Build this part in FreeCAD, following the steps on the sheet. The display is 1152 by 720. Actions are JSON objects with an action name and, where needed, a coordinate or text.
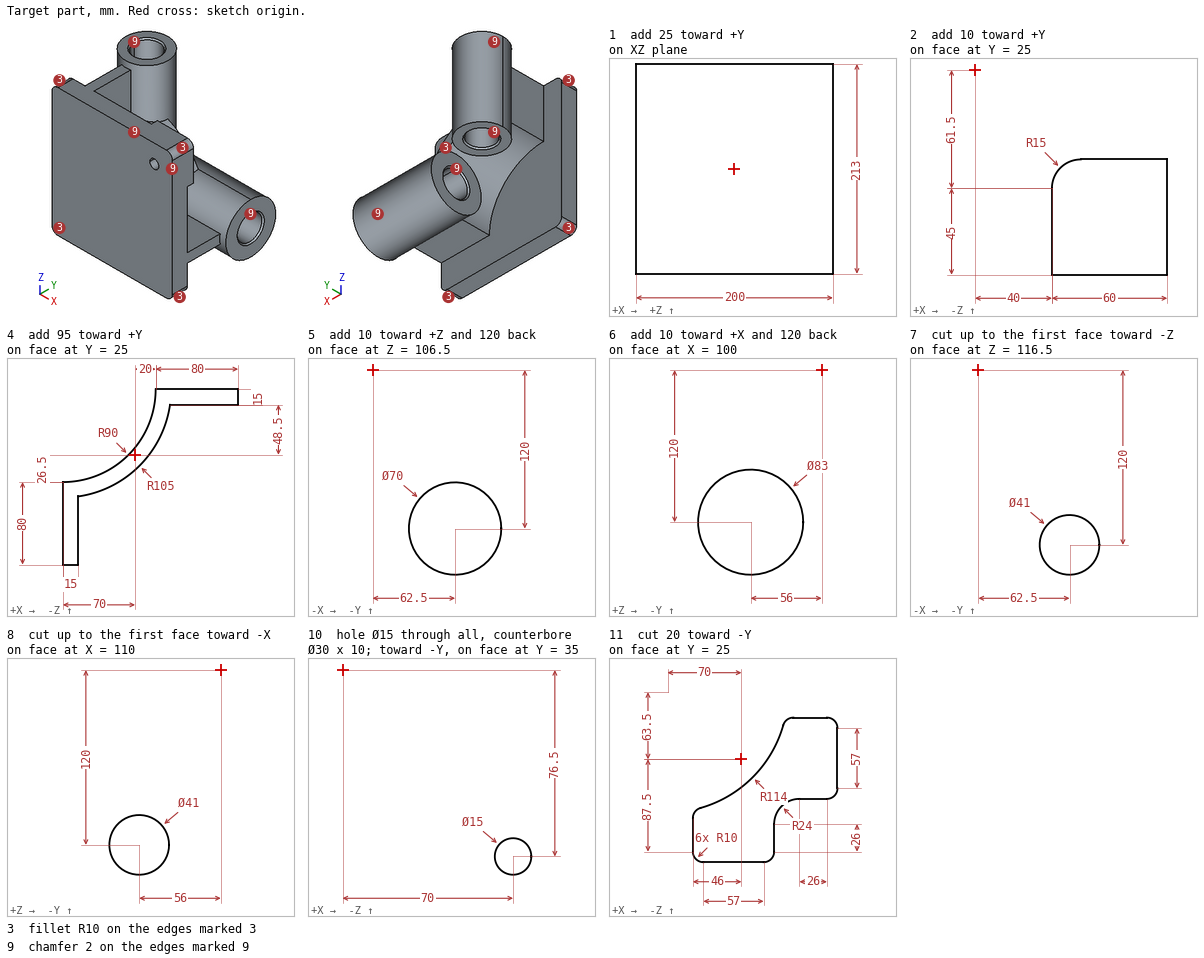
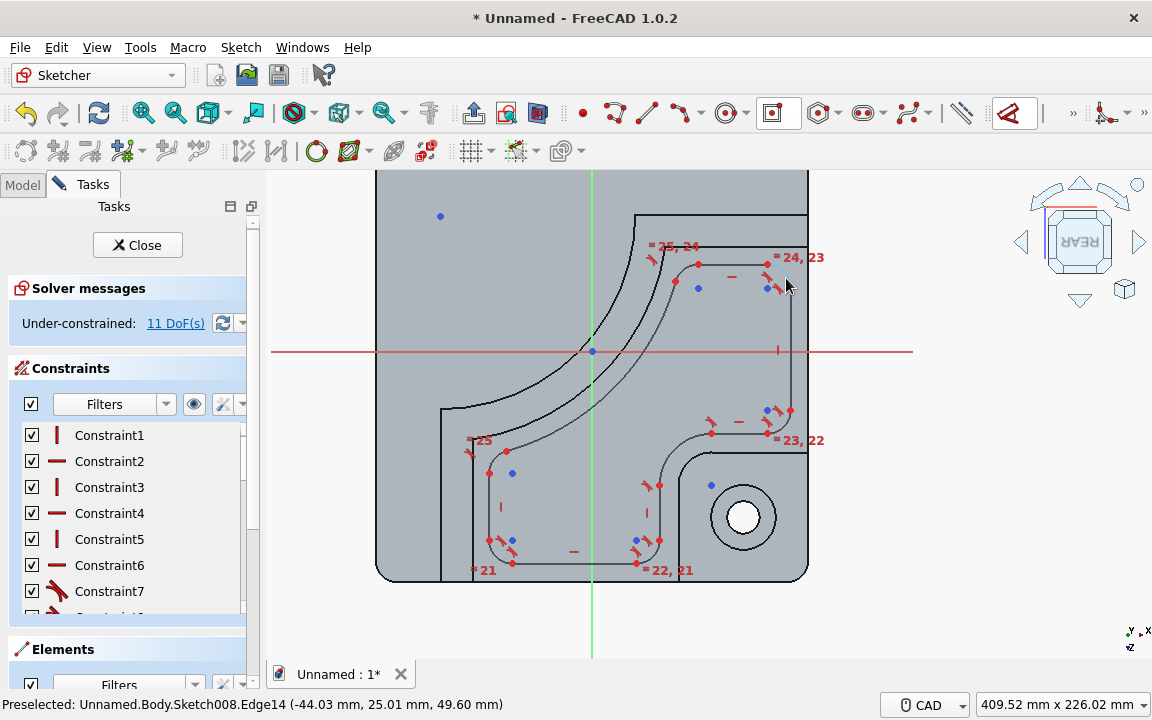
{"action": "scroll", "coordinate": [492, 551], "scroll_direction": "up", "scroll_amount": 4}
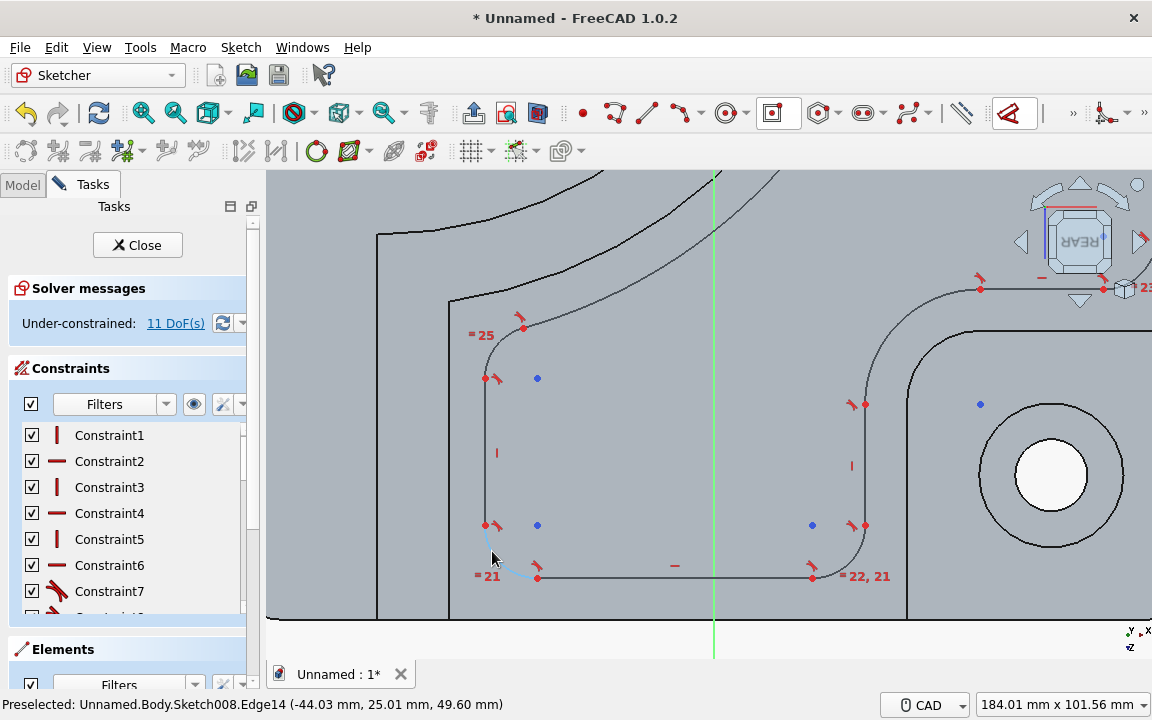
{"action": "left_click", "coordinate": [491, 549]}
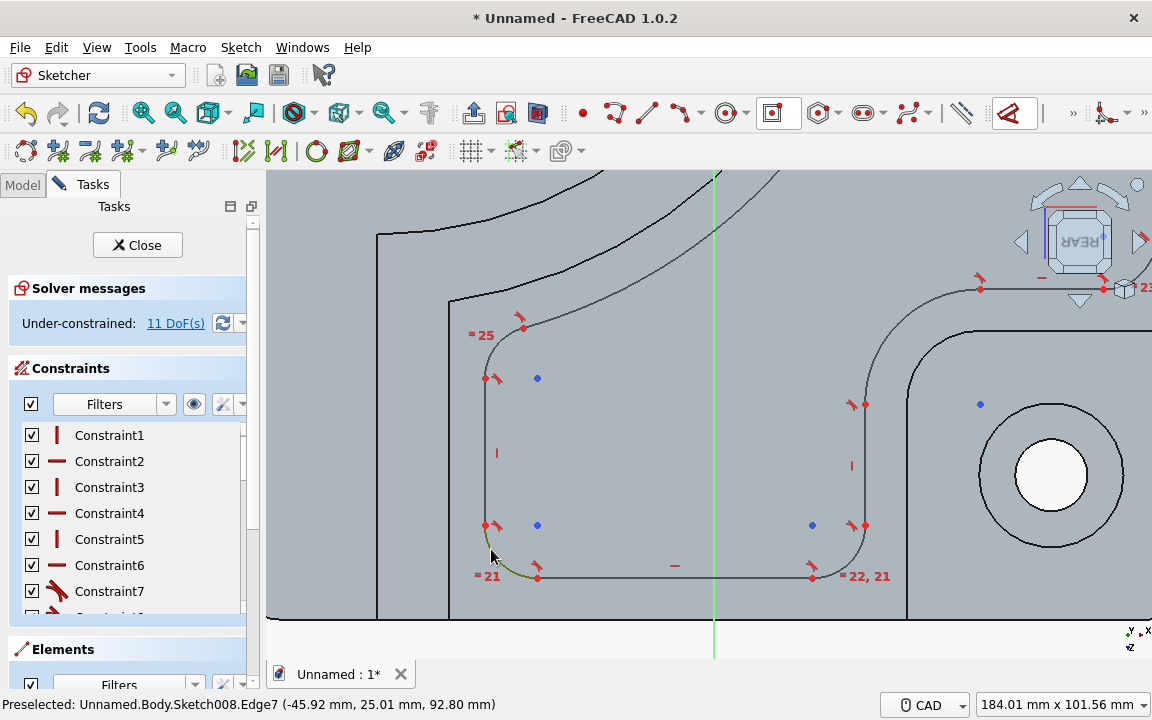
{"action": "key", "text": "k r"}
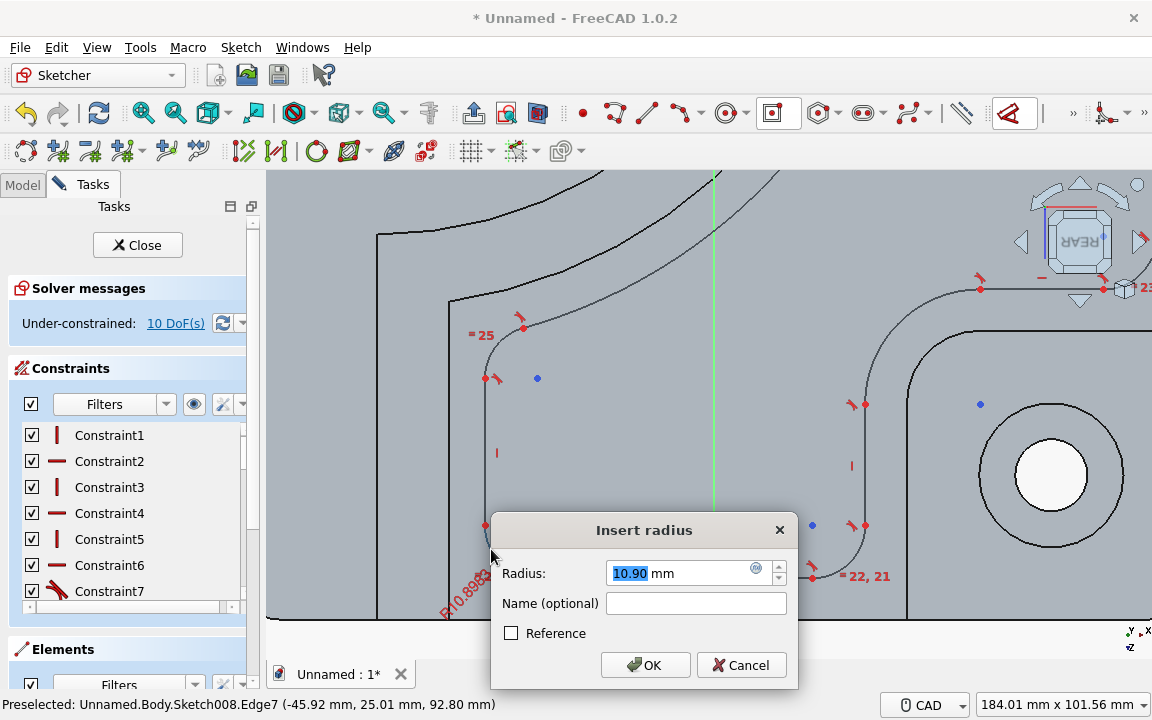
{"action": "type", "text": "10"}
{"action": "key", "text": "Return"}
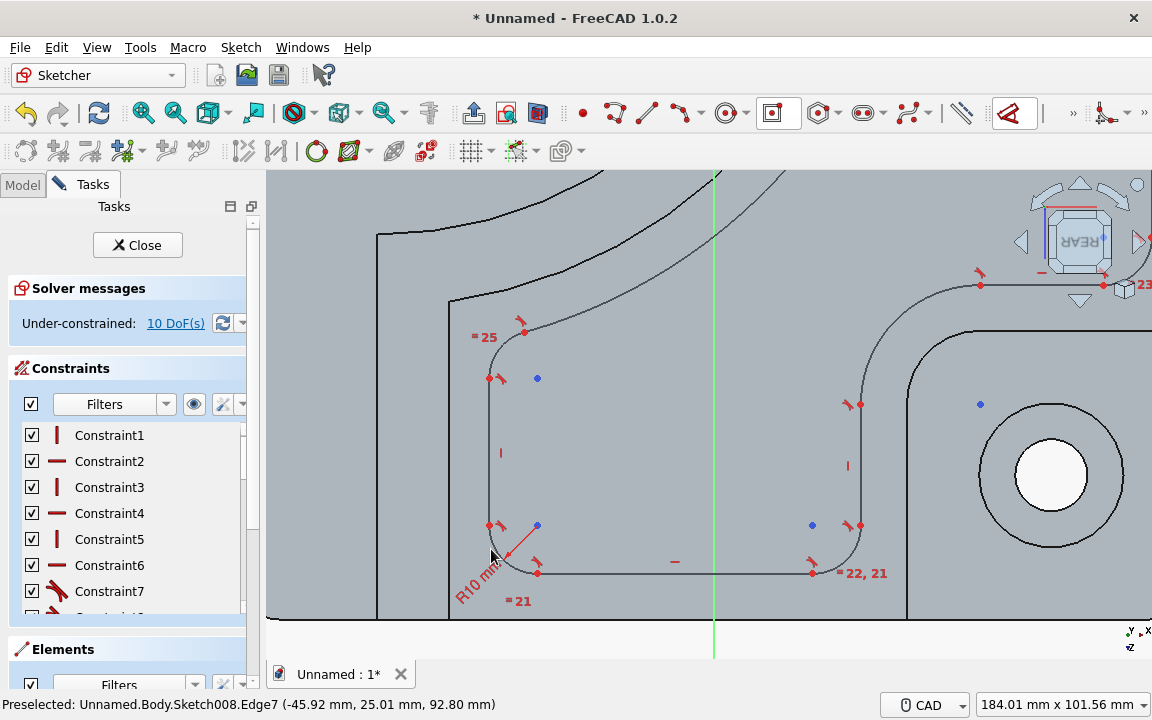
{"action": "left_click", "coordinate": [926, 298]}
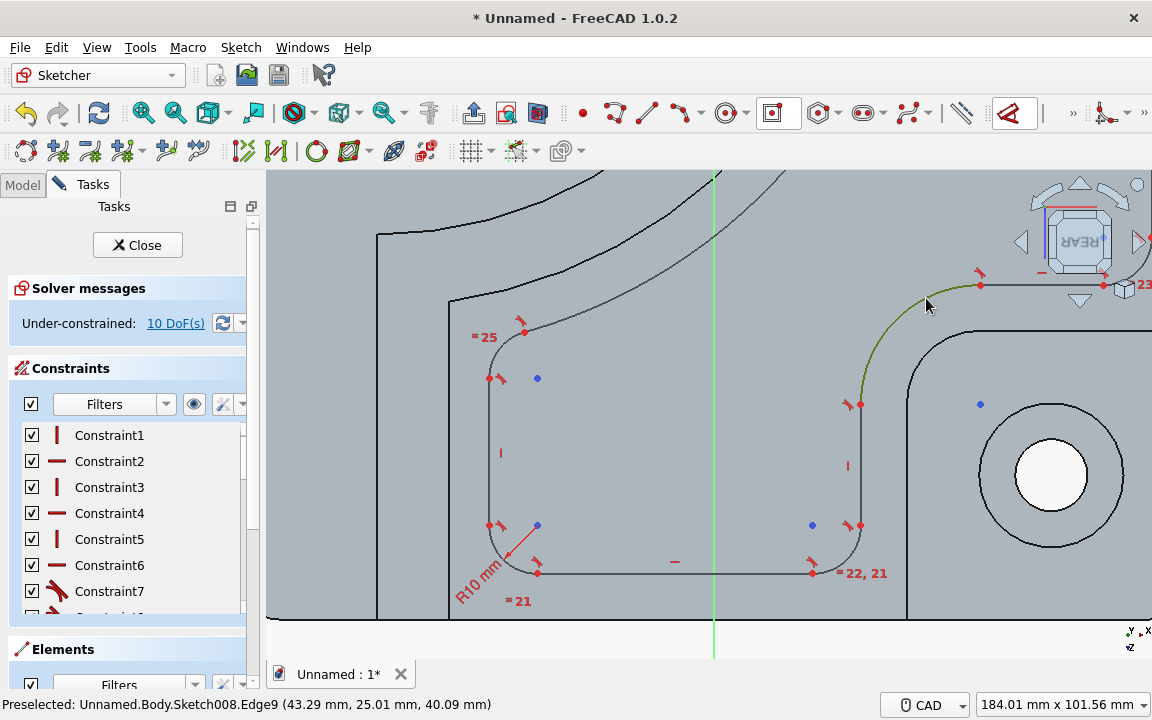
{"action": "left_click", "coordinate": [1032, 114]}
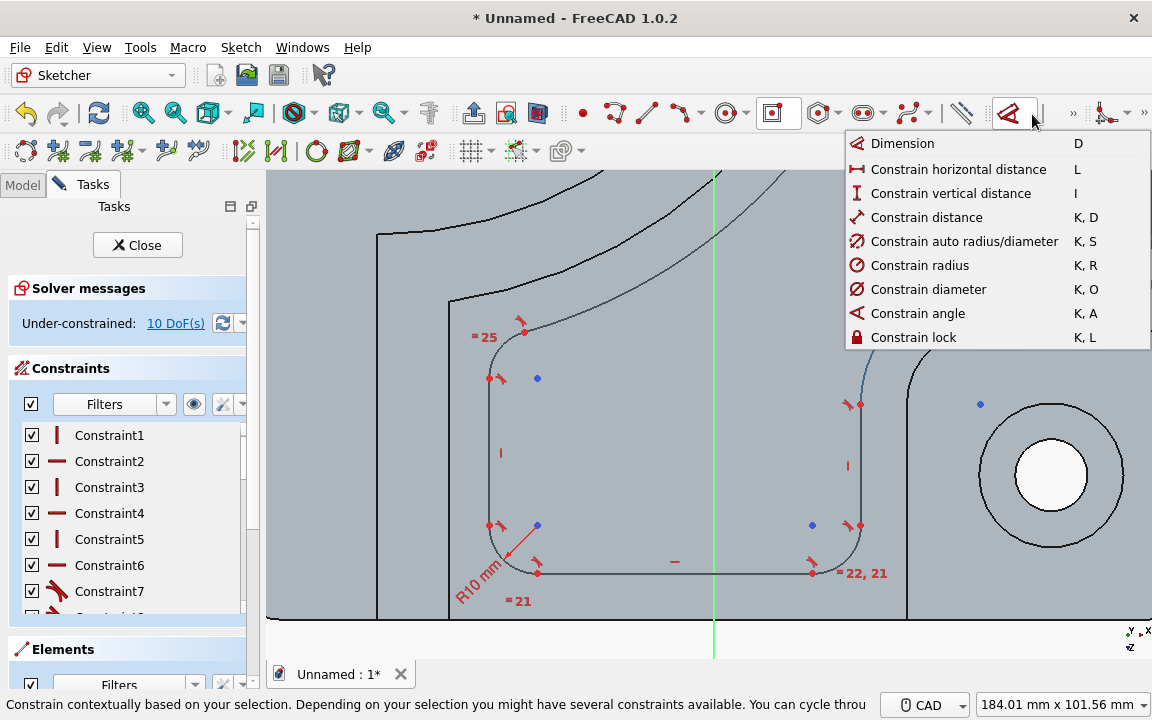
{"action": "left_click", "coordinate": [998, 265]}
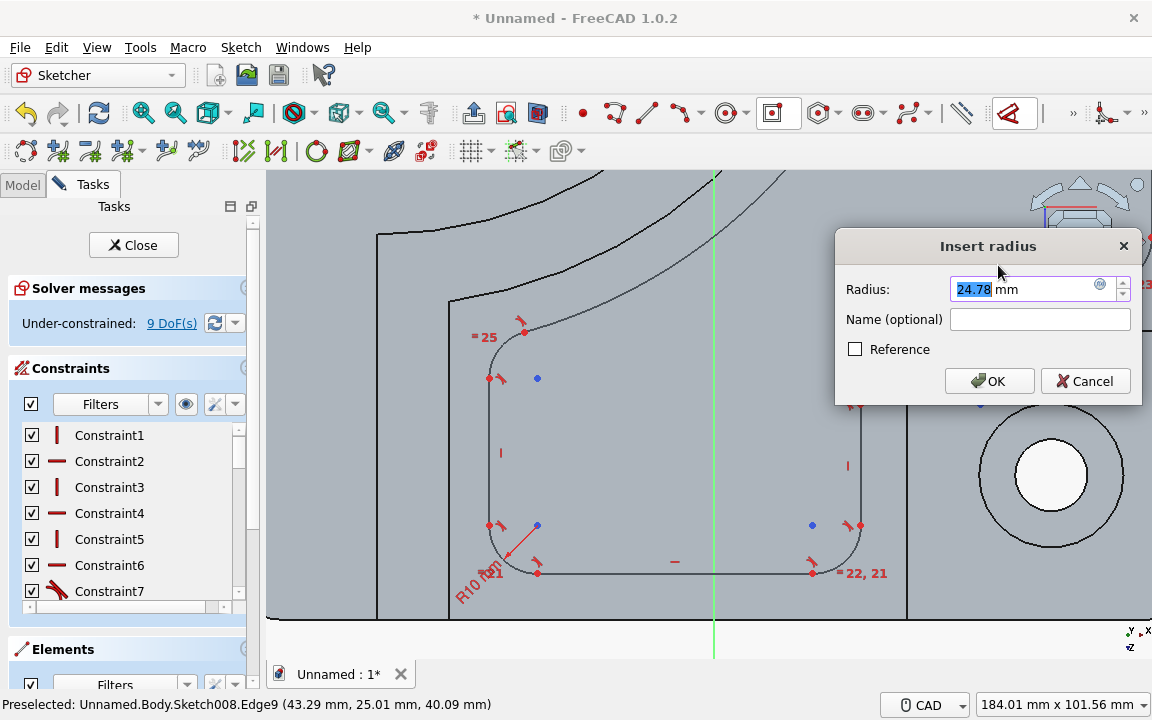
{"action": "type", "text": "24"}
{"action": "key", "text": "Return"}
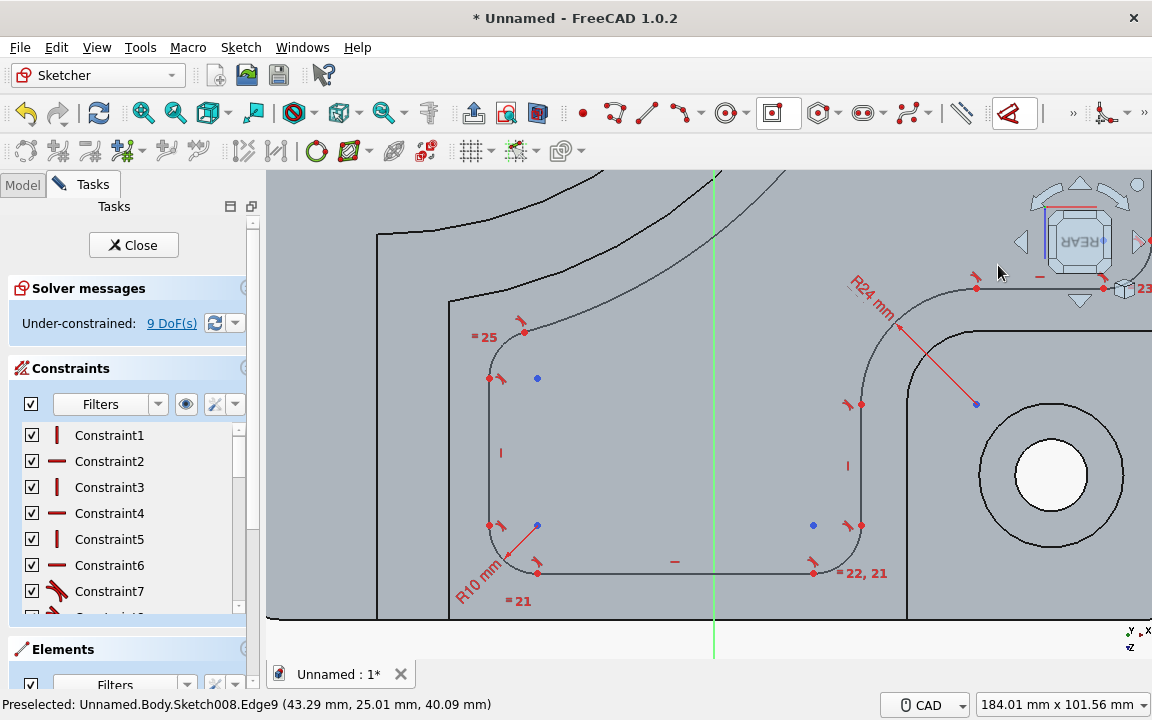
{"action": "left_click", "coordinate": [678, 263]}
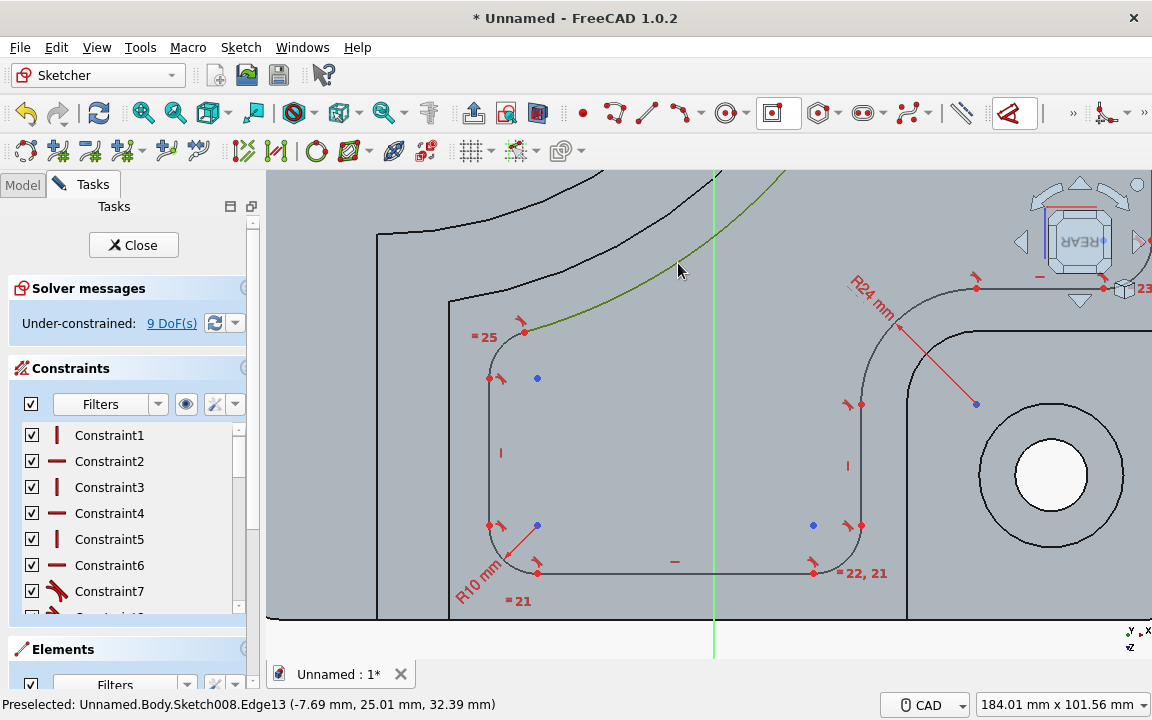
{"action": "left_click", "coordinate": [1032, 114]}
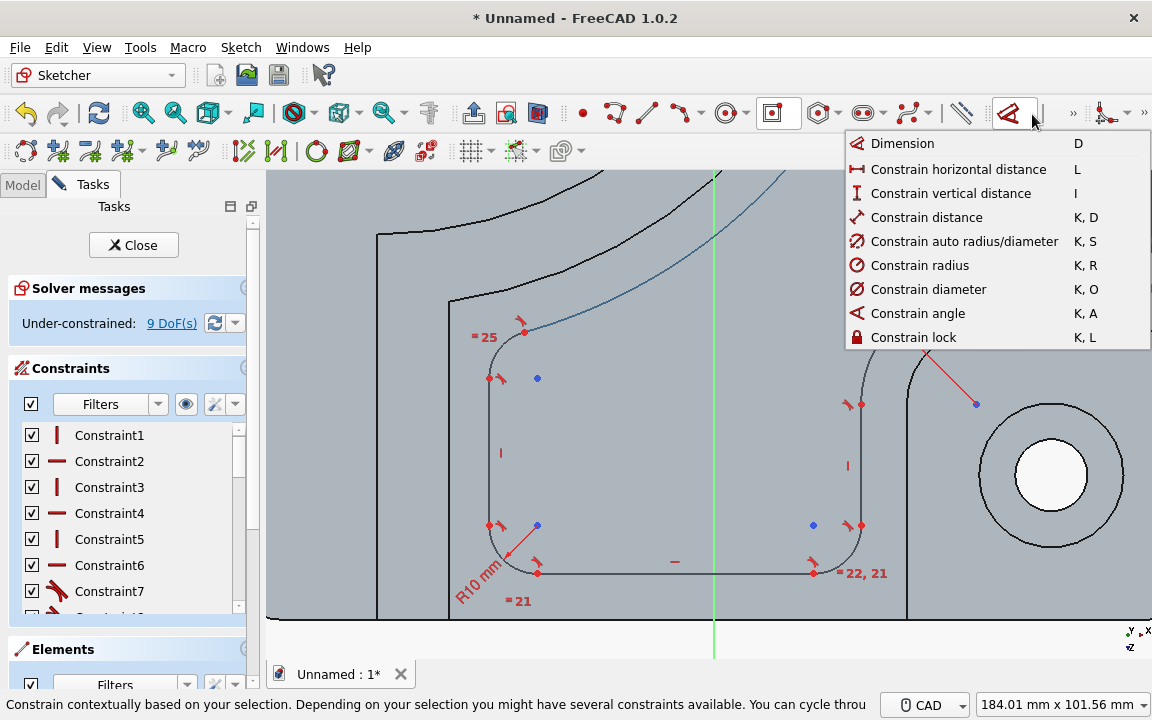
{"action": "left_click", "coordinate": [998, 265]}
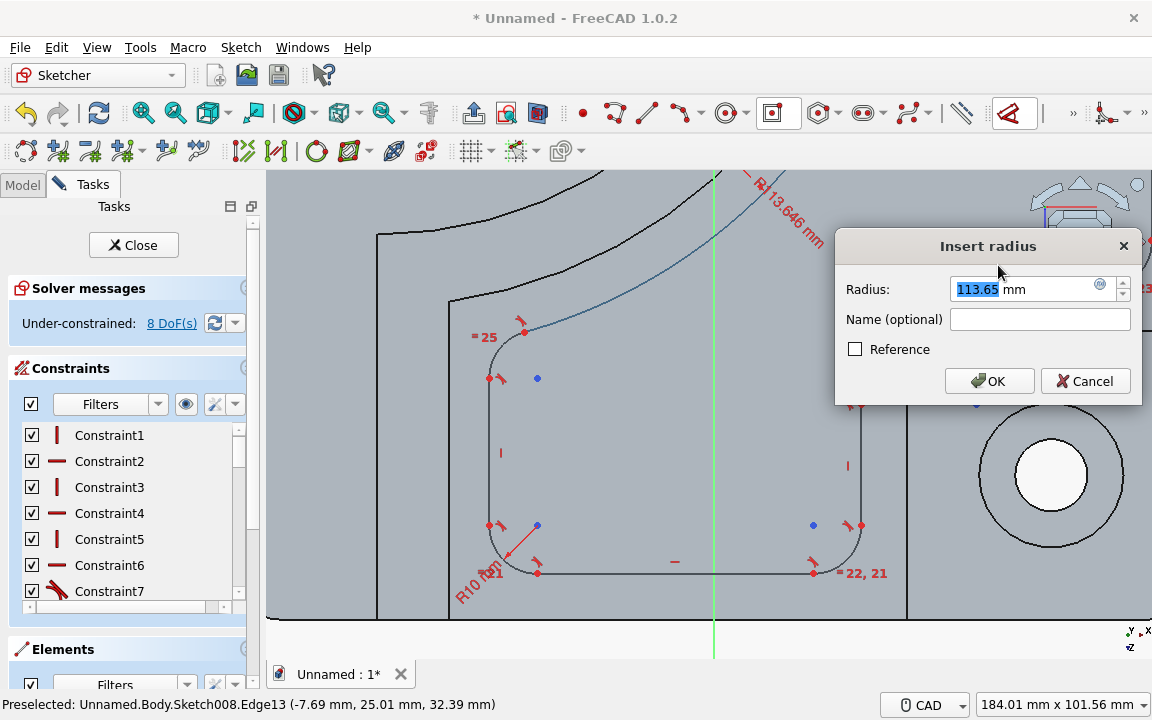
{"action": "type", "text": "114"}
{"action": "key", "text": "Return"}